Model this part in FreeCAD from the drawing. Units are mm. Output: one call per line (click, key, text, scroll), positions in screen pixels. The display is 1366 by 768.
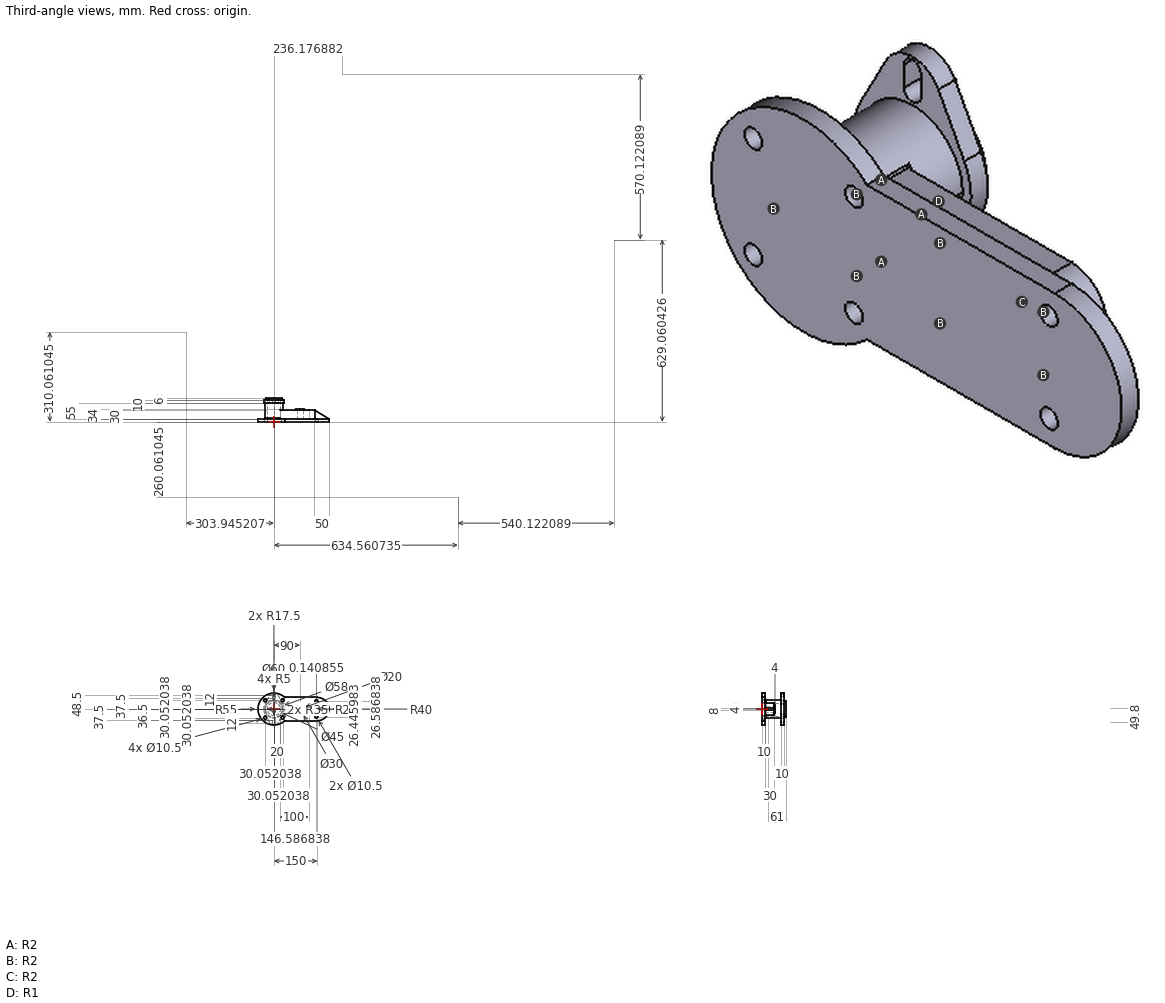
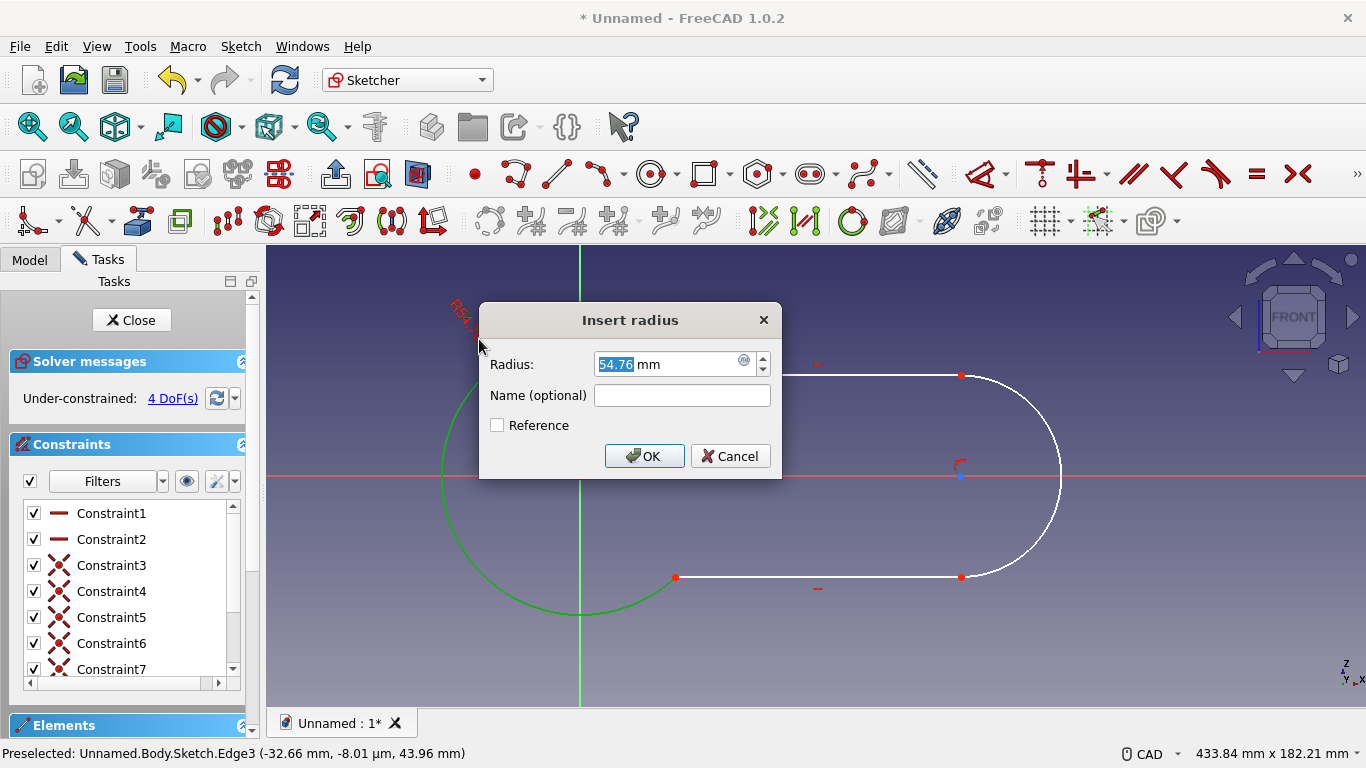
text(55)
key(Return)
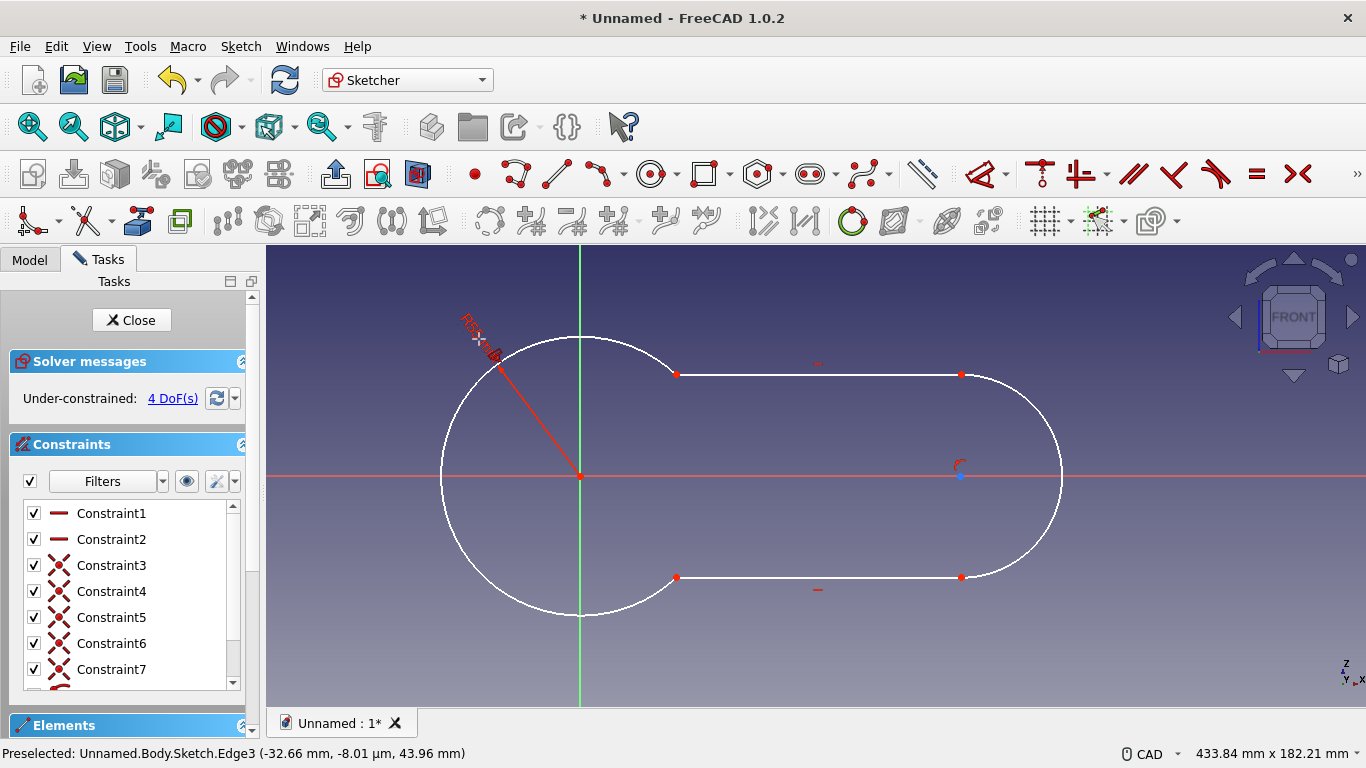
click(1043, 536)
click(1069, 555)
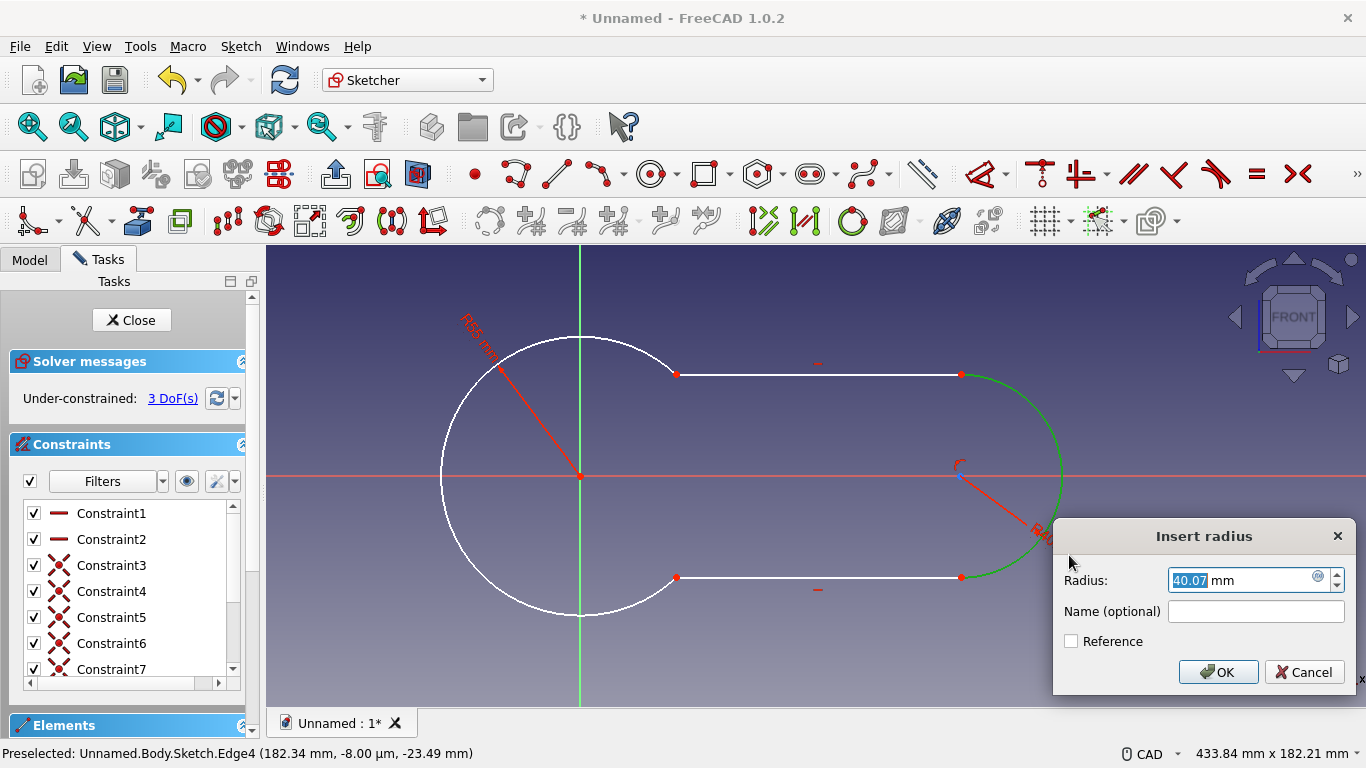
text(40)
key(Return)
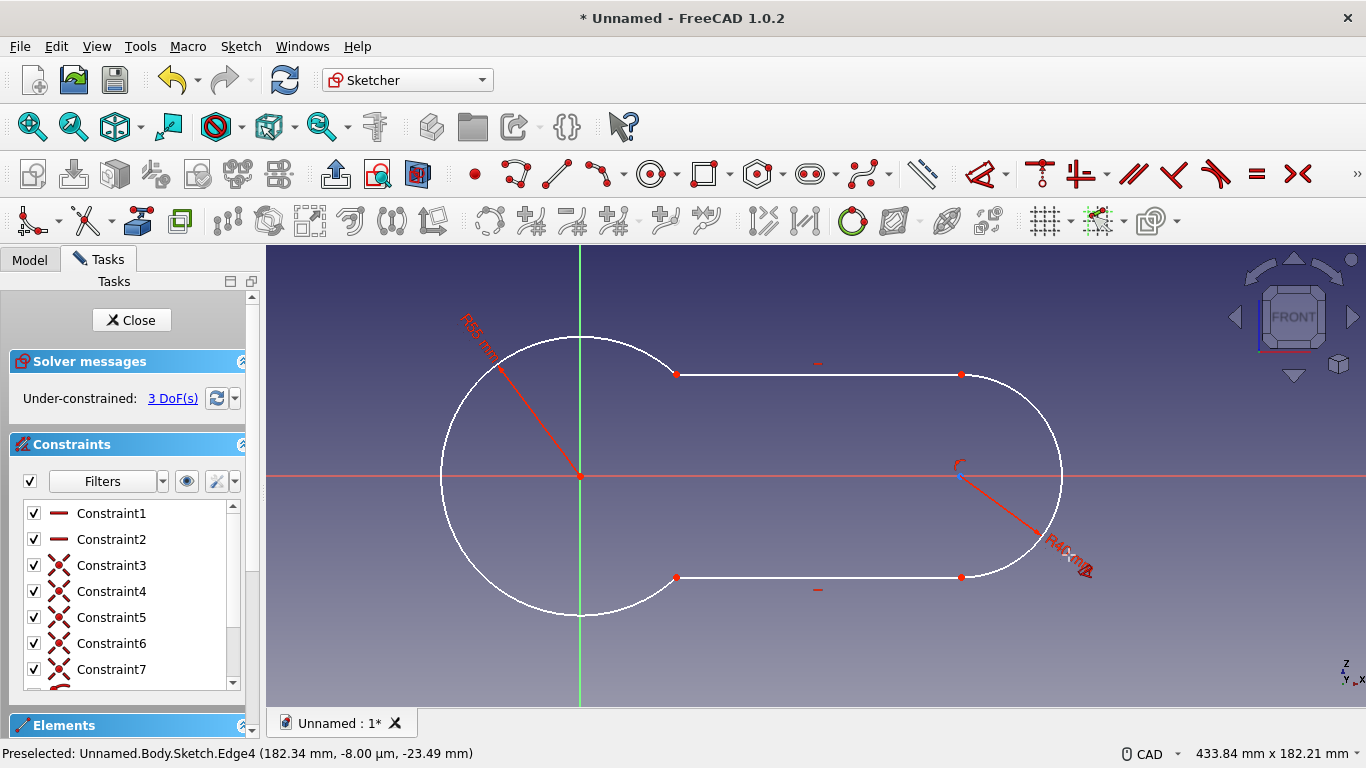
click(961, 578)
click(771, 612)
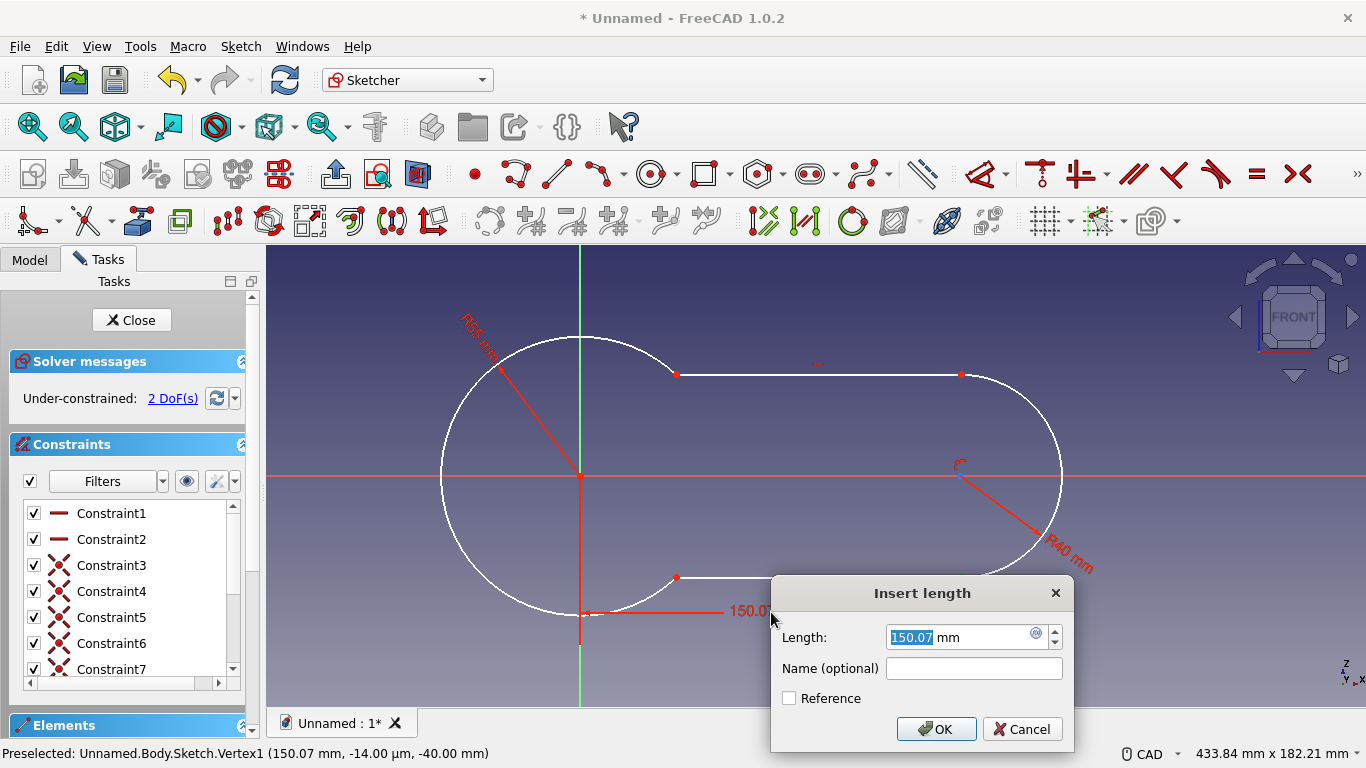
text(150)
key(Return)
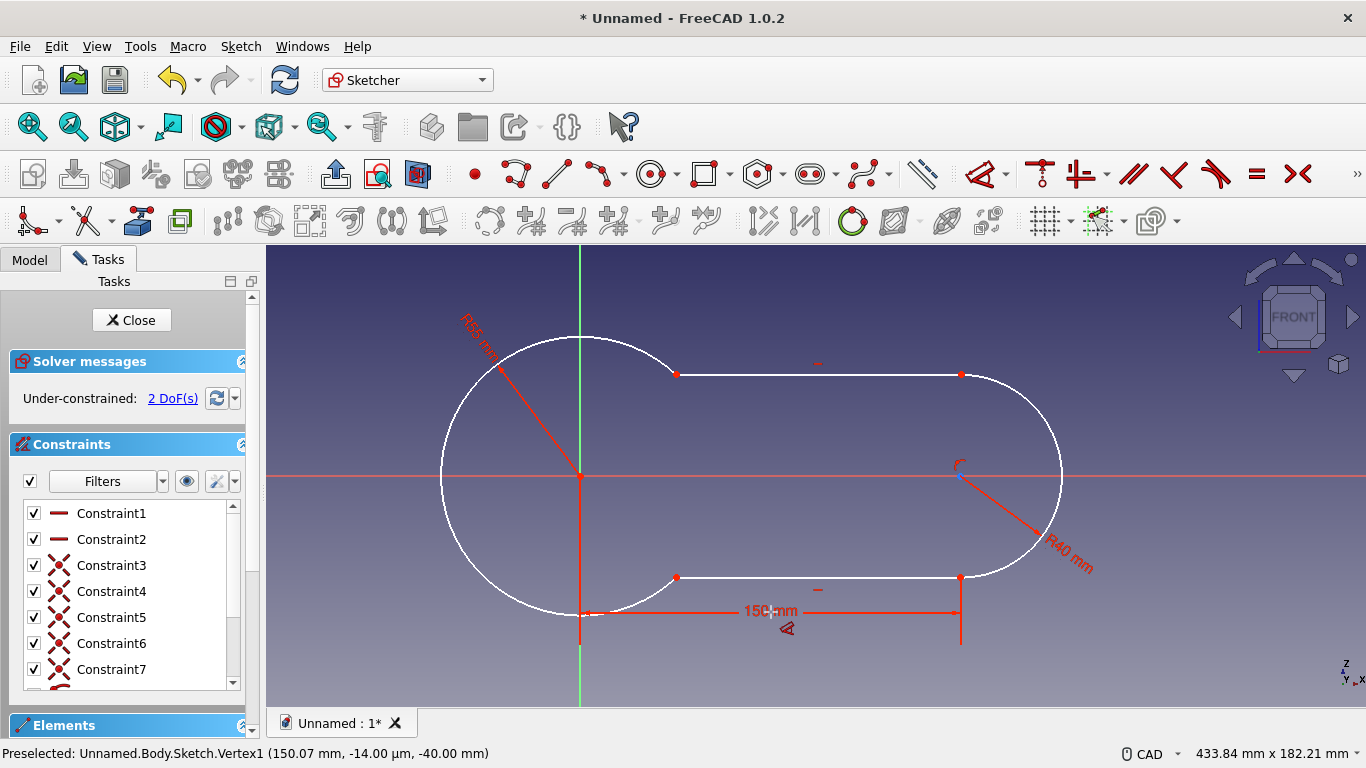
click(961, 375)
click(771, 341)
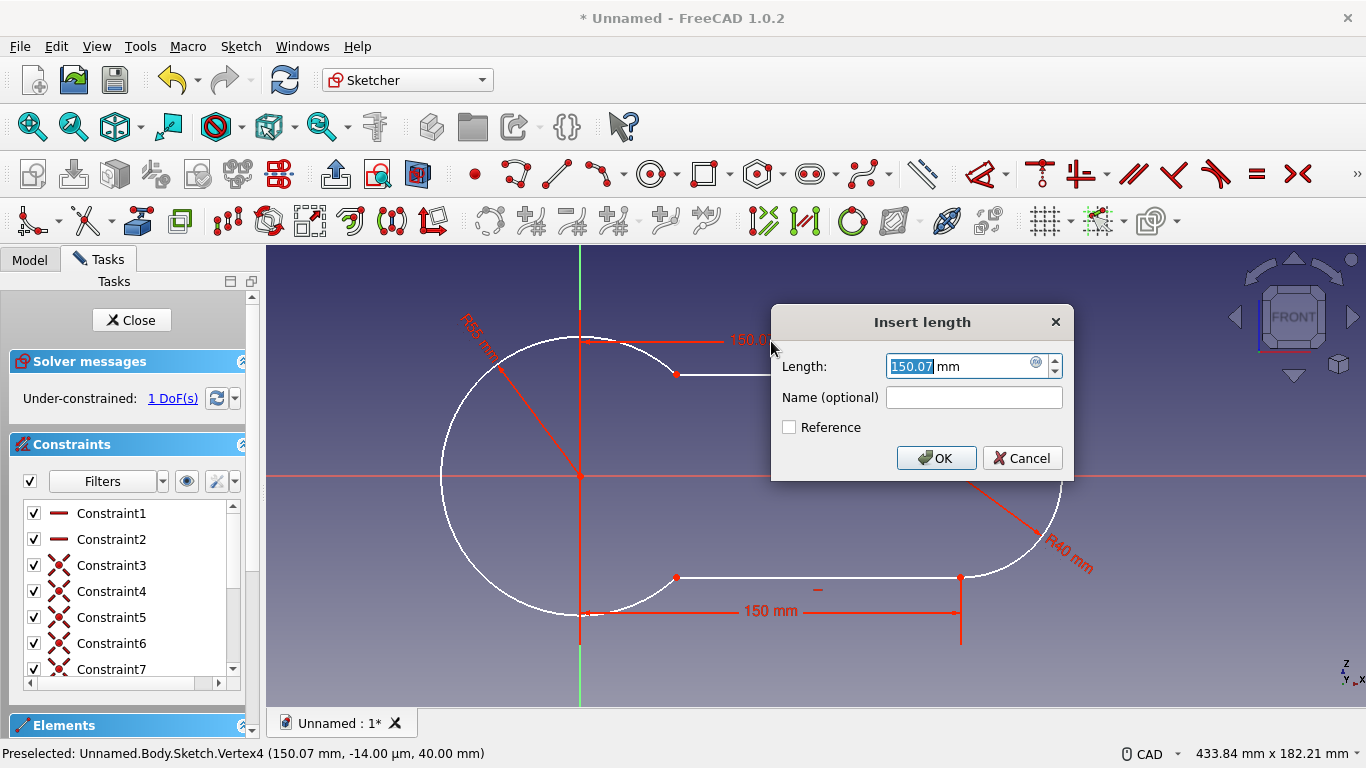
text(150)
key(Return)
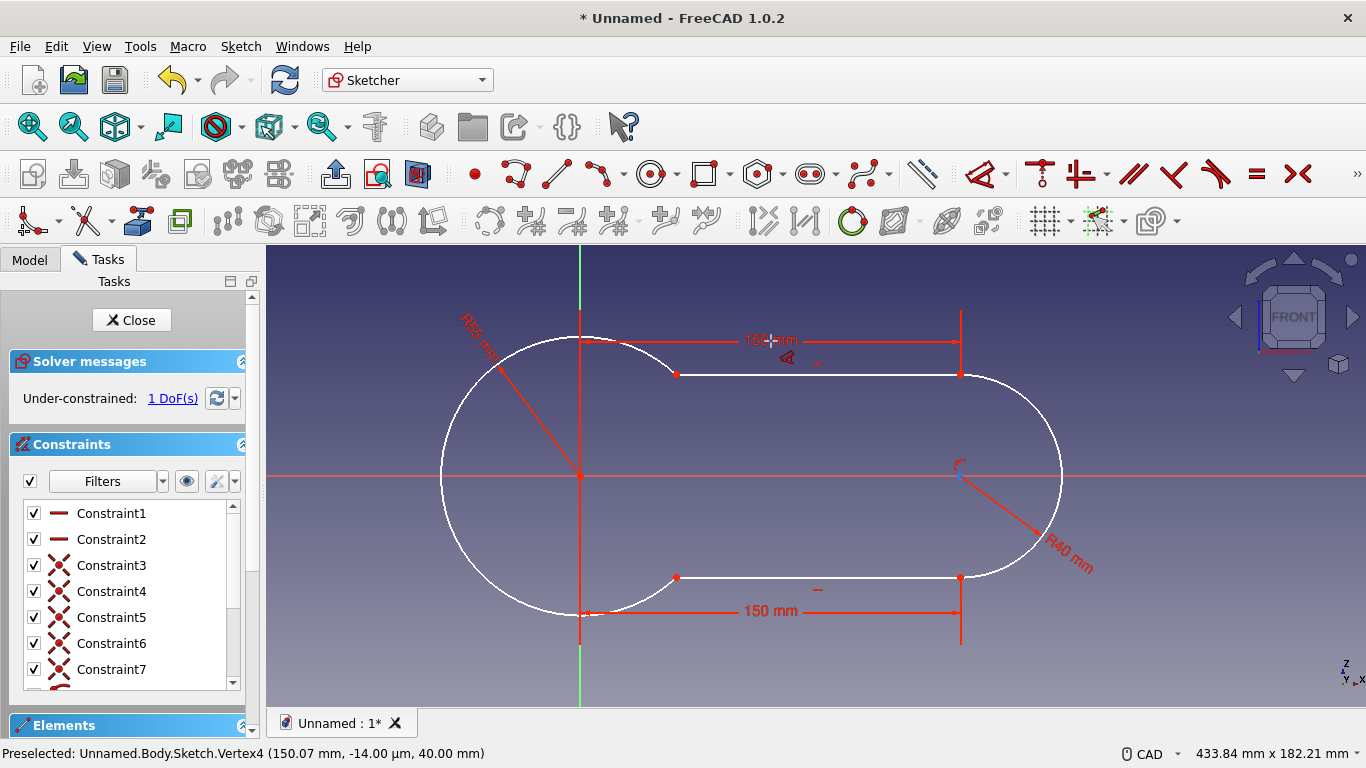
click(961, 476)
click(771, 510)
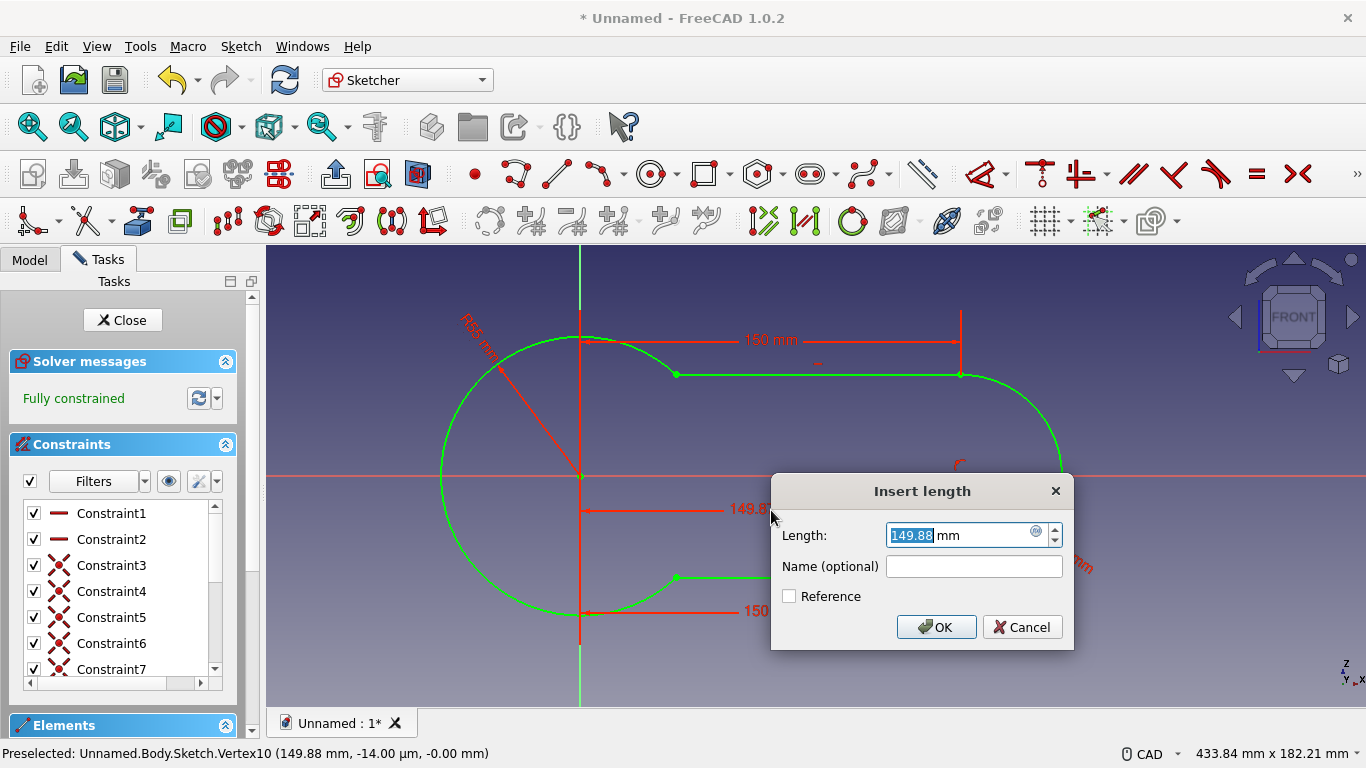
text(150)
key(Return)
key(Escape)